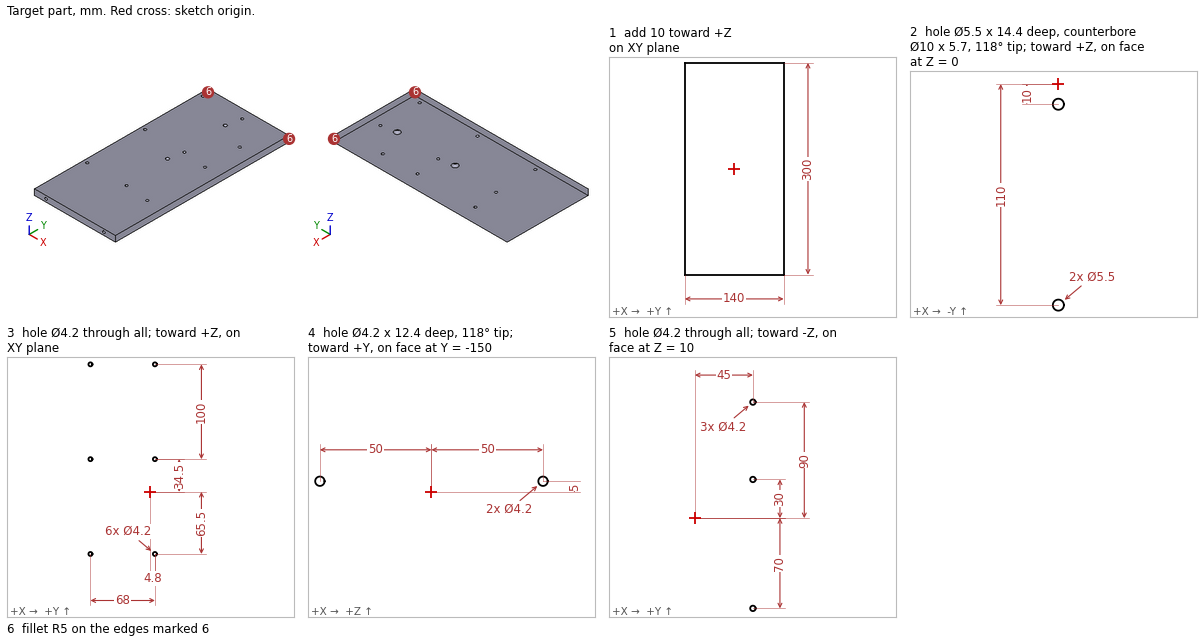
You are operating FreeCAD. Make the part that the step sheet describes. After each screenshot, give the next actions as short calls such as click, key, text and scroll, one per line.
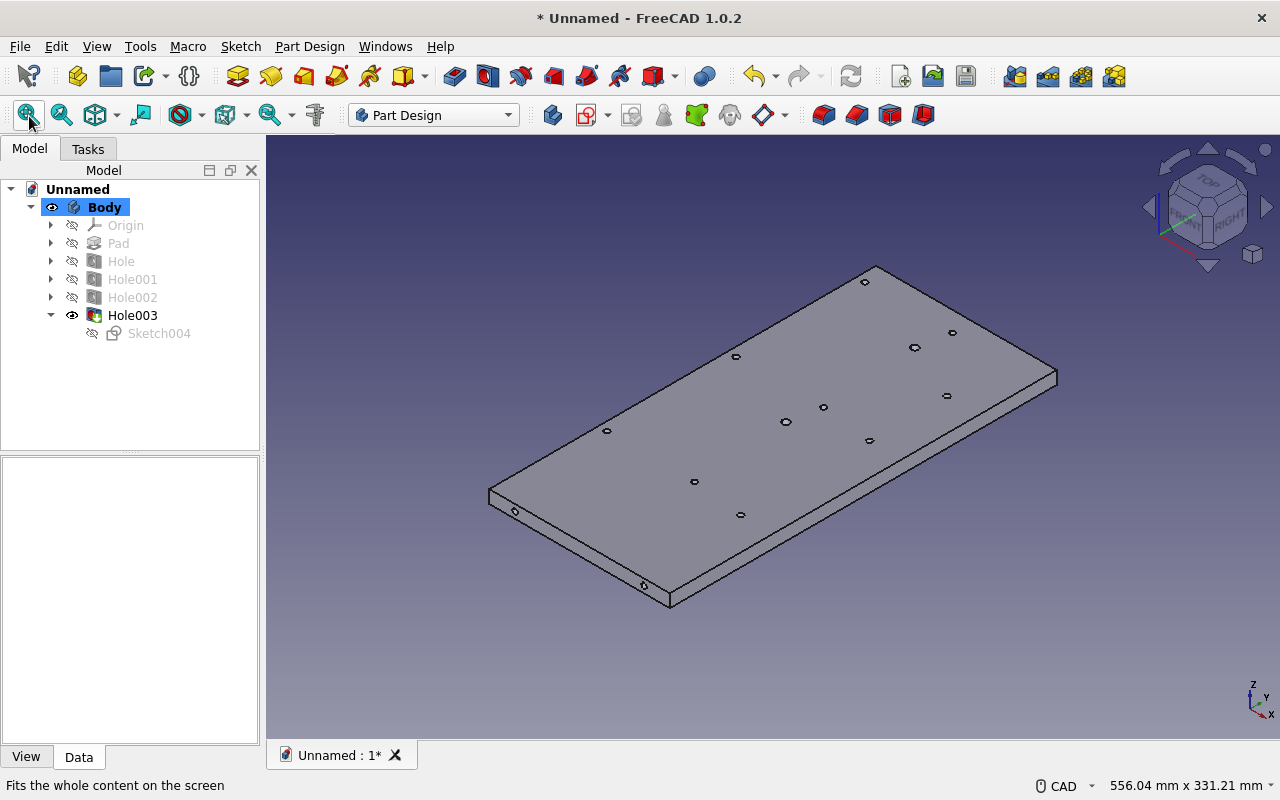
key(2)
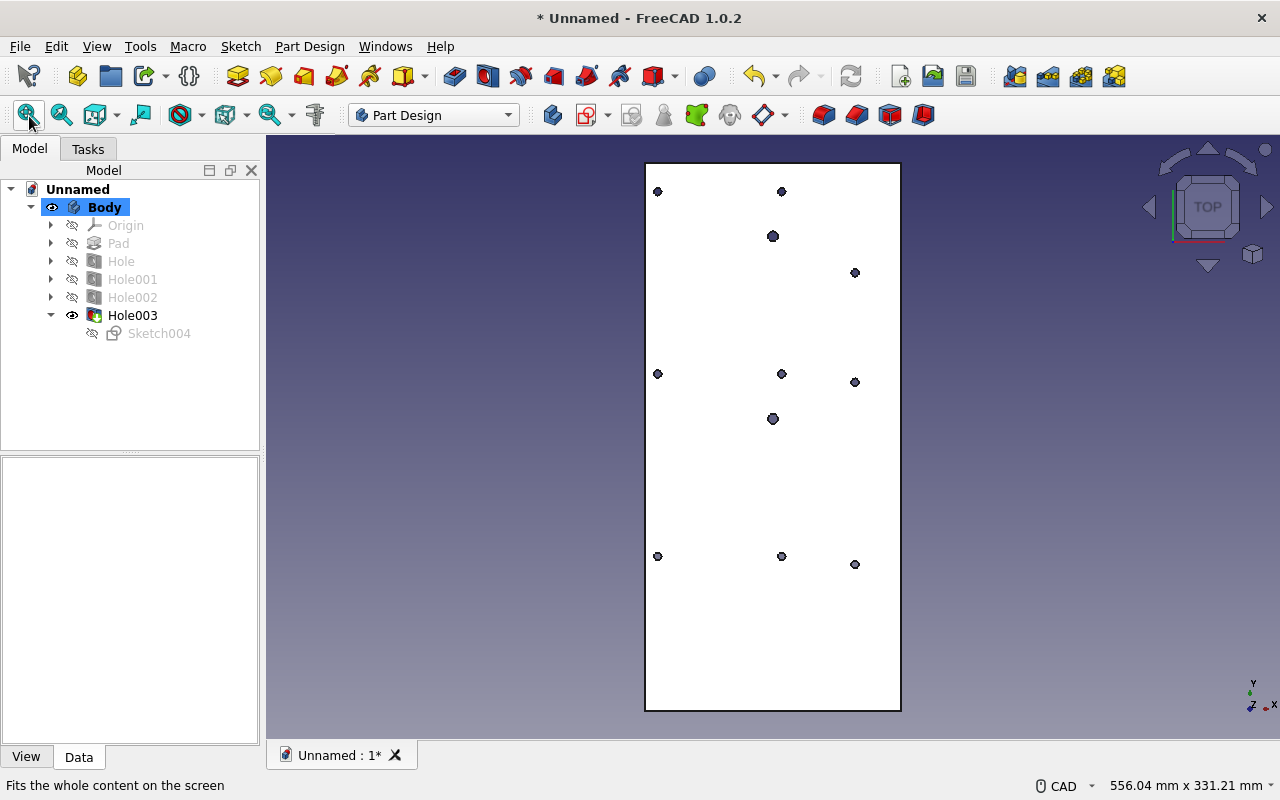
key(0)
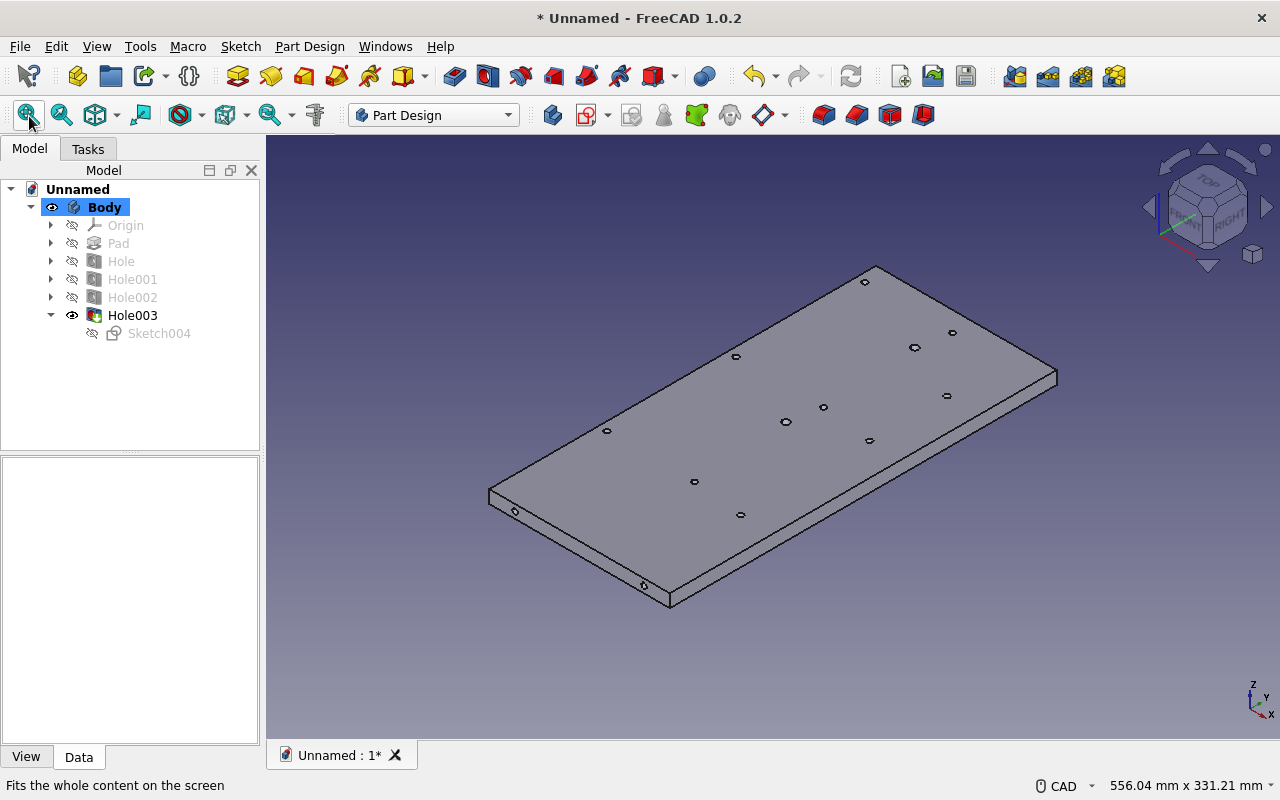
scroll(876, 272, up, 4)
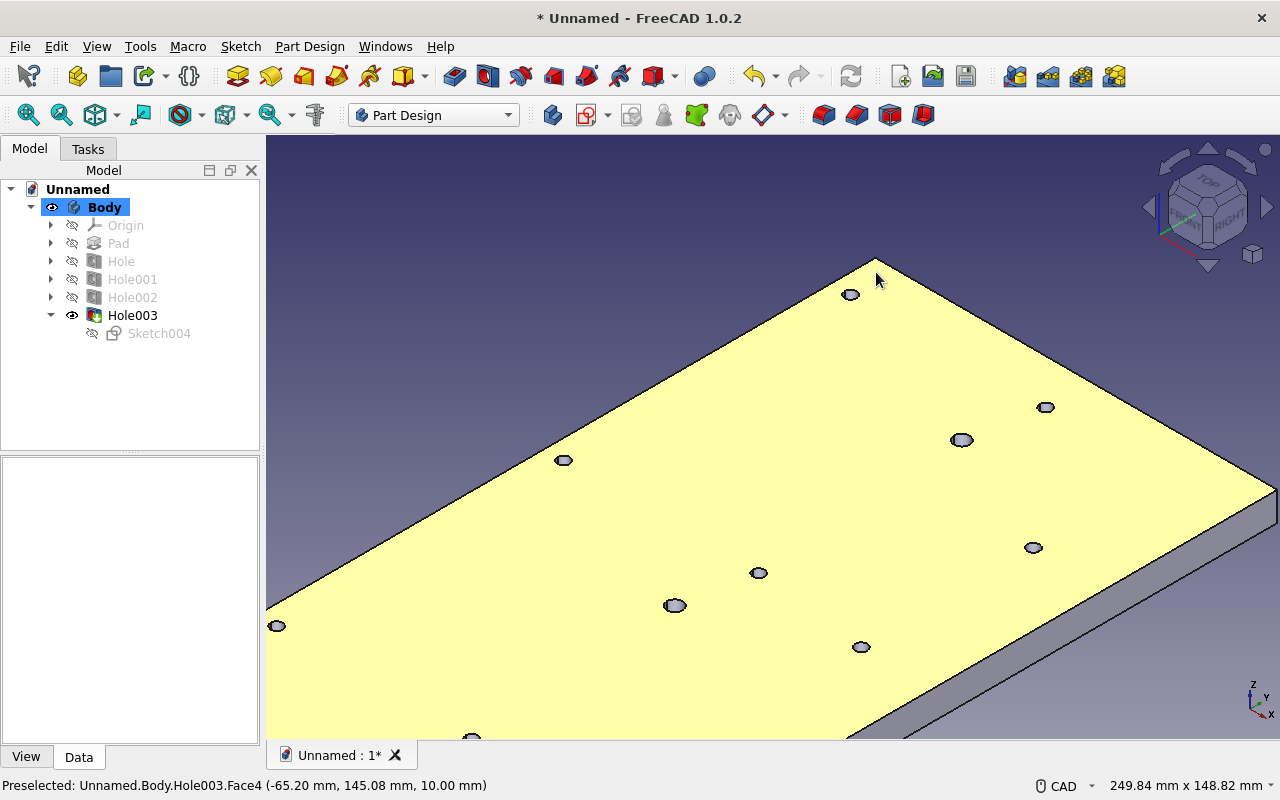
click(29, 116)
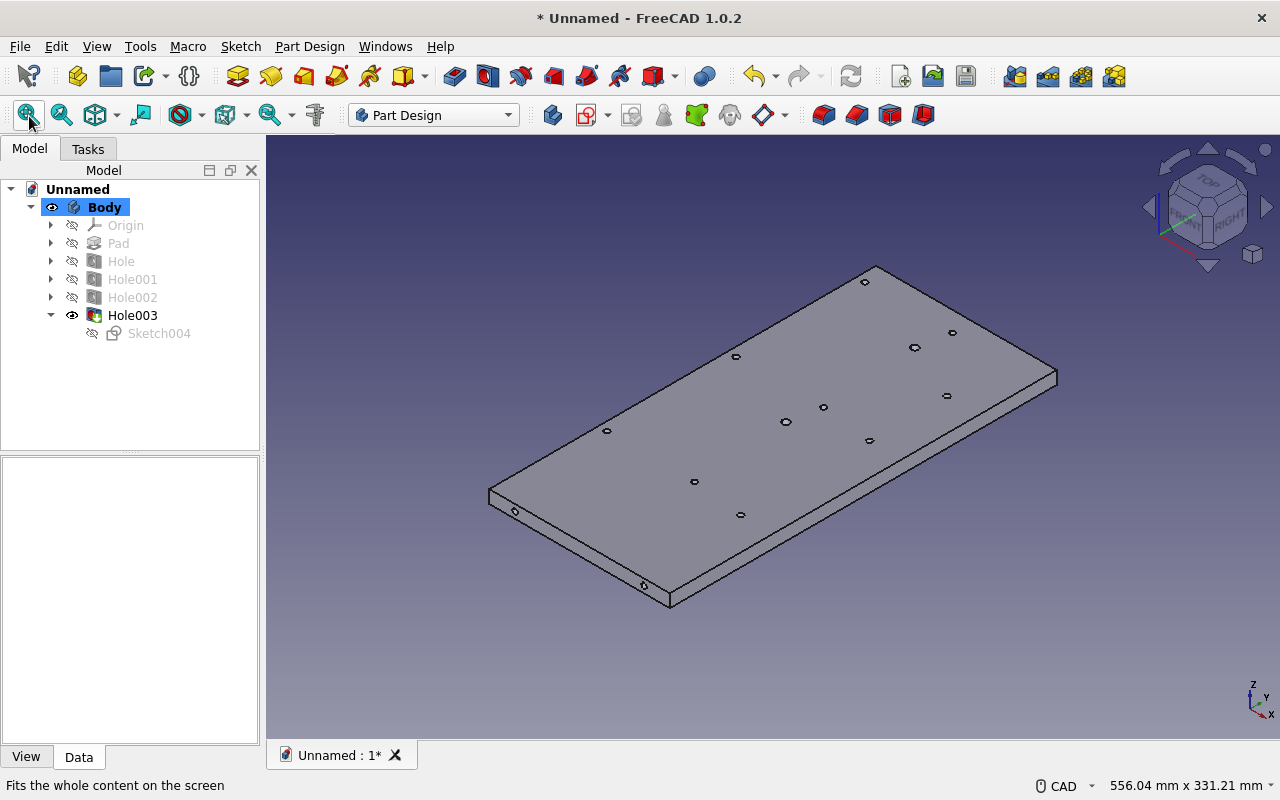
key(1)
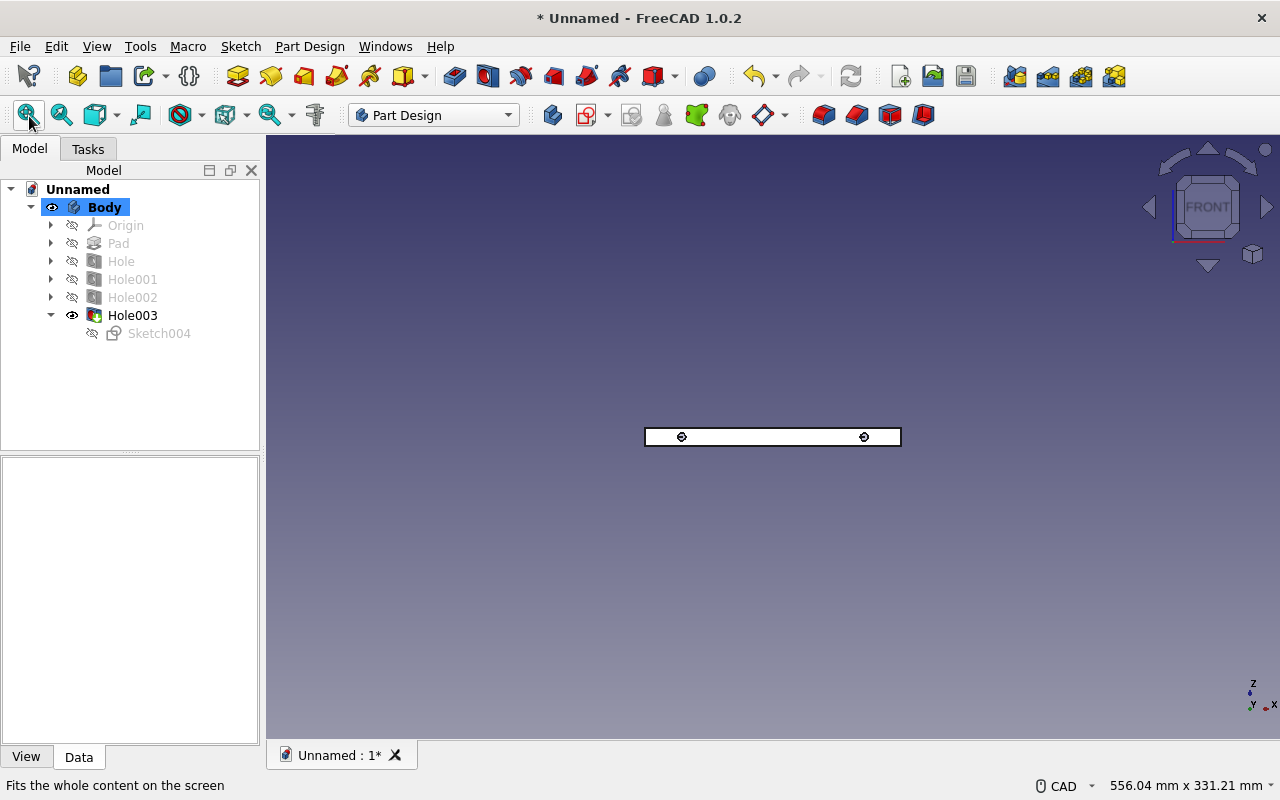
key(v)
key(f)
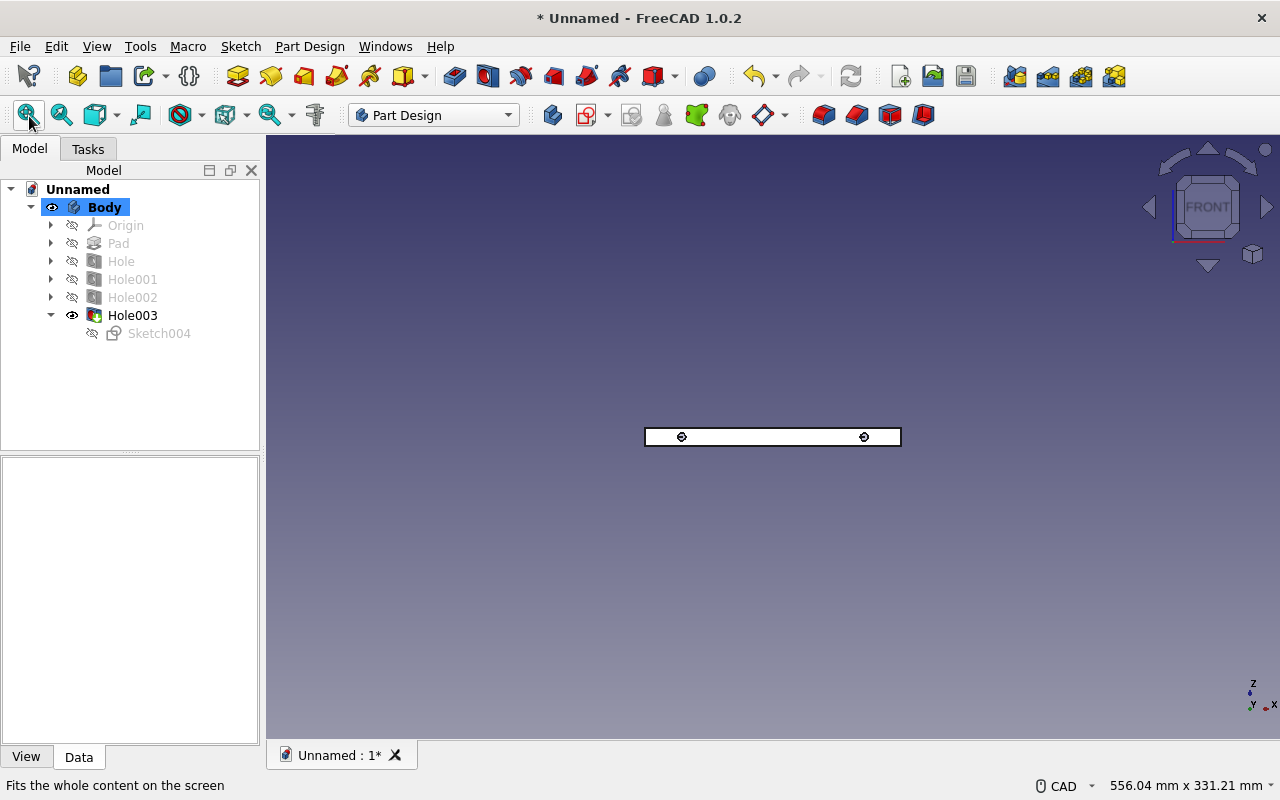
scroll(645, 436, up, 4)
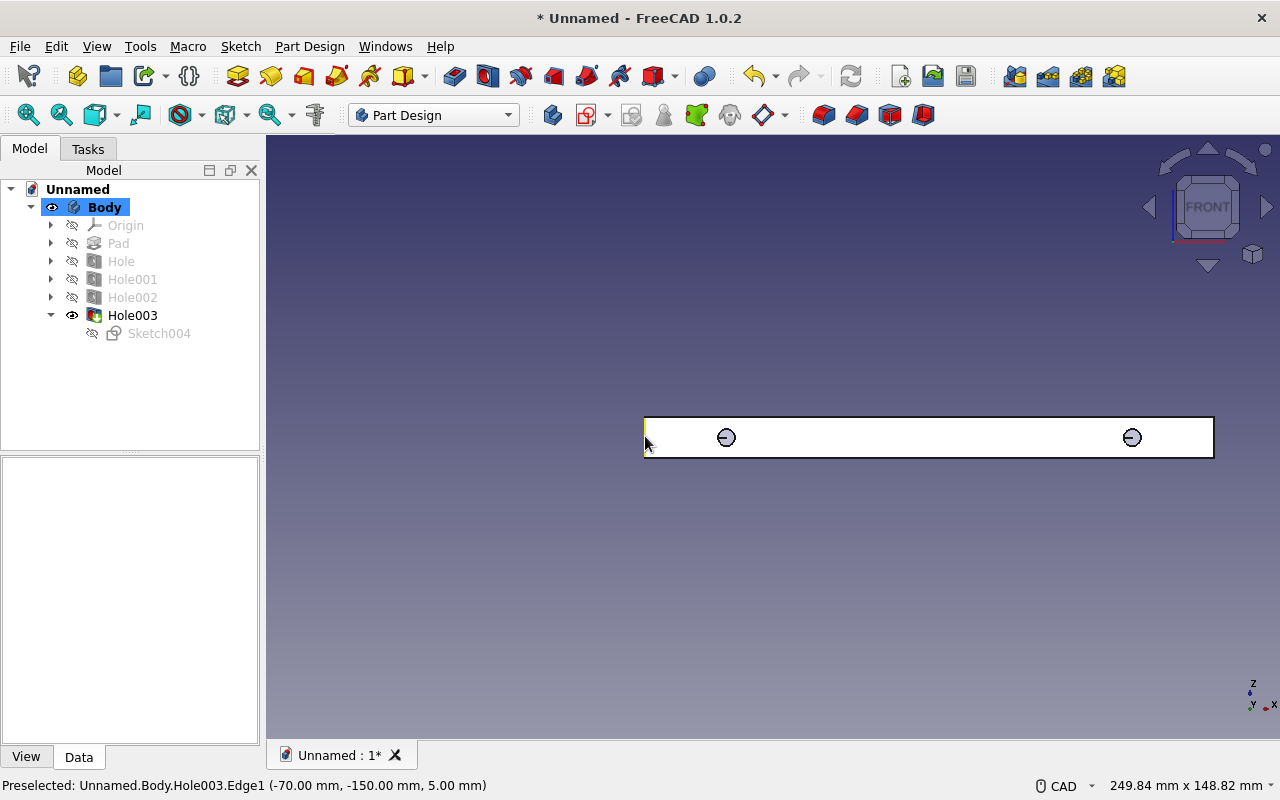
click(29, 116)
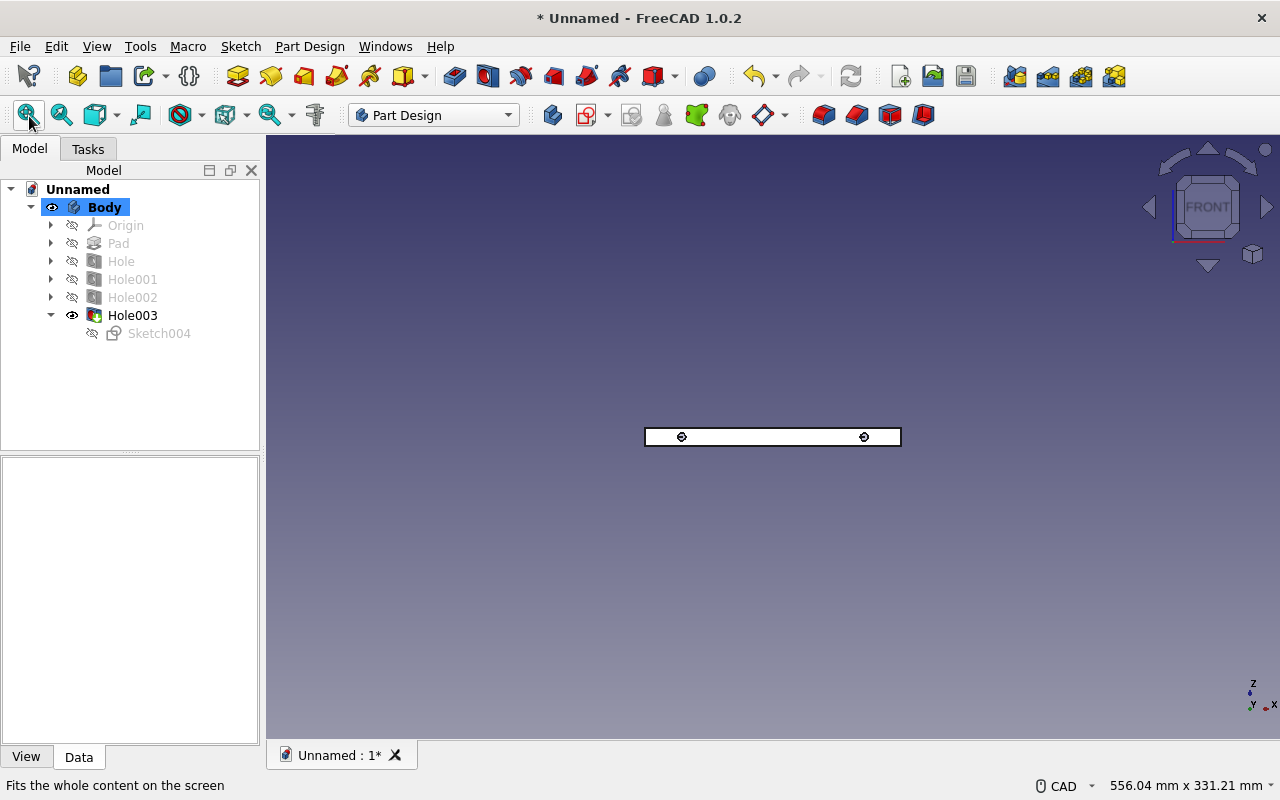
key(3)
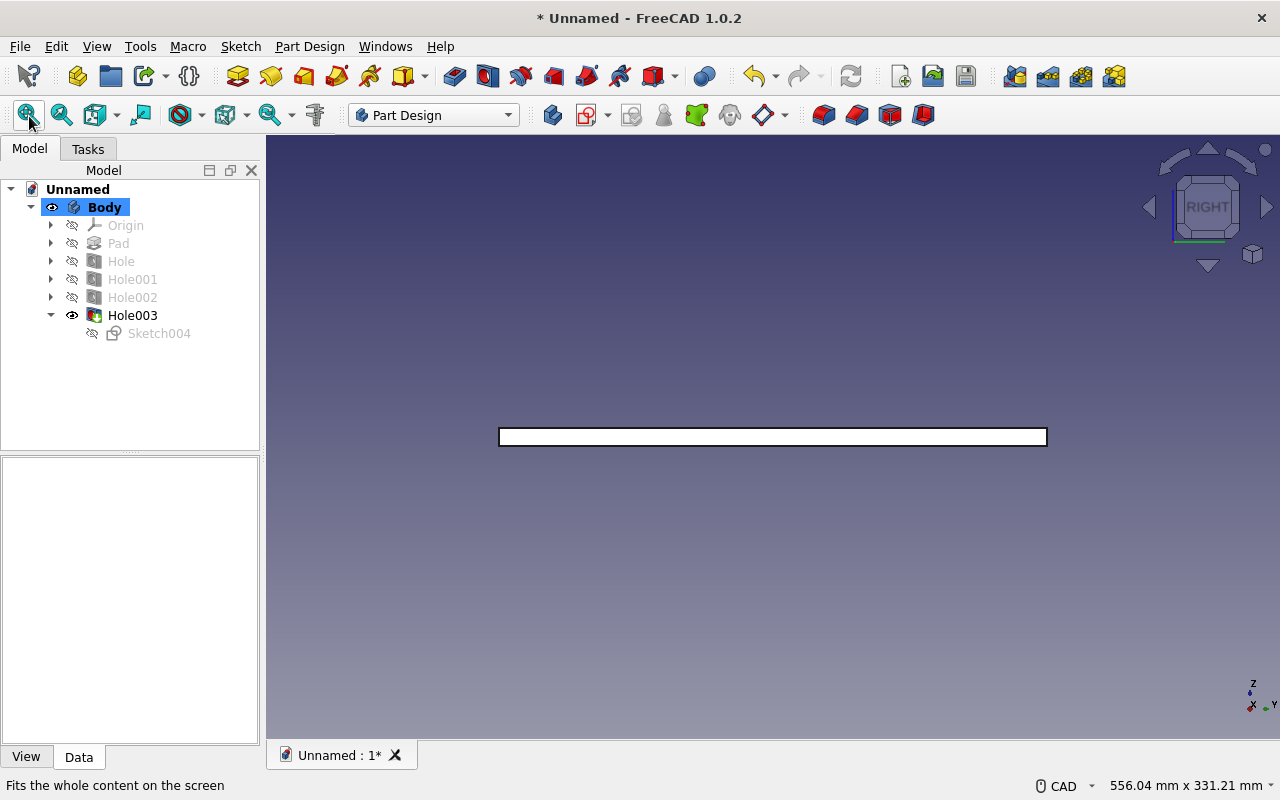
click(1047, 436)